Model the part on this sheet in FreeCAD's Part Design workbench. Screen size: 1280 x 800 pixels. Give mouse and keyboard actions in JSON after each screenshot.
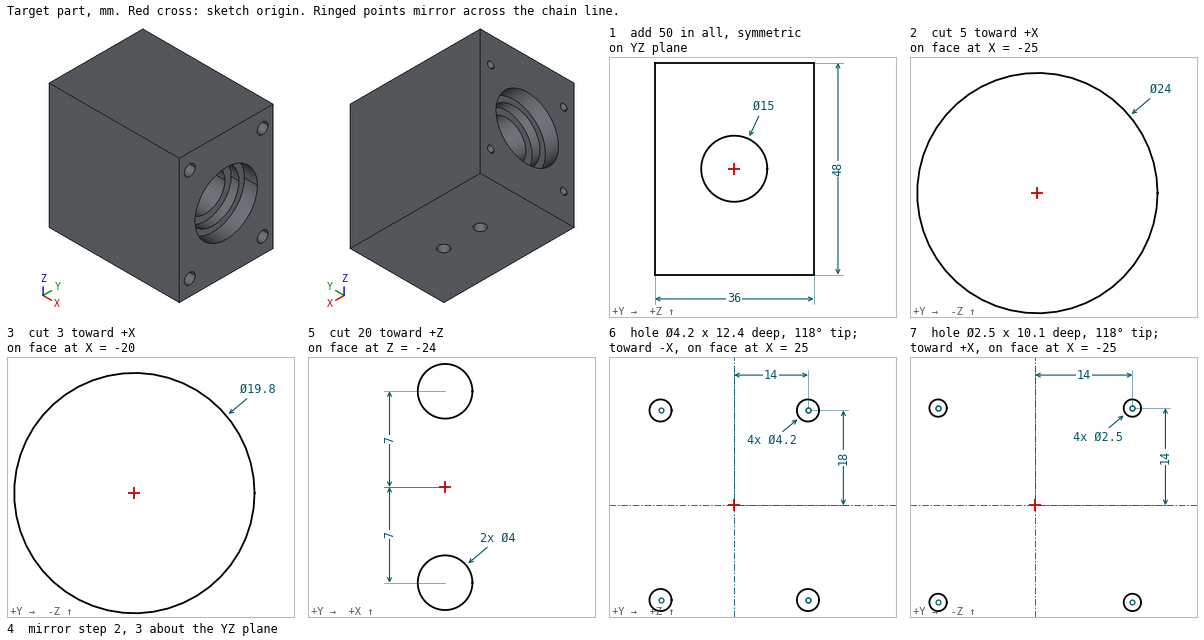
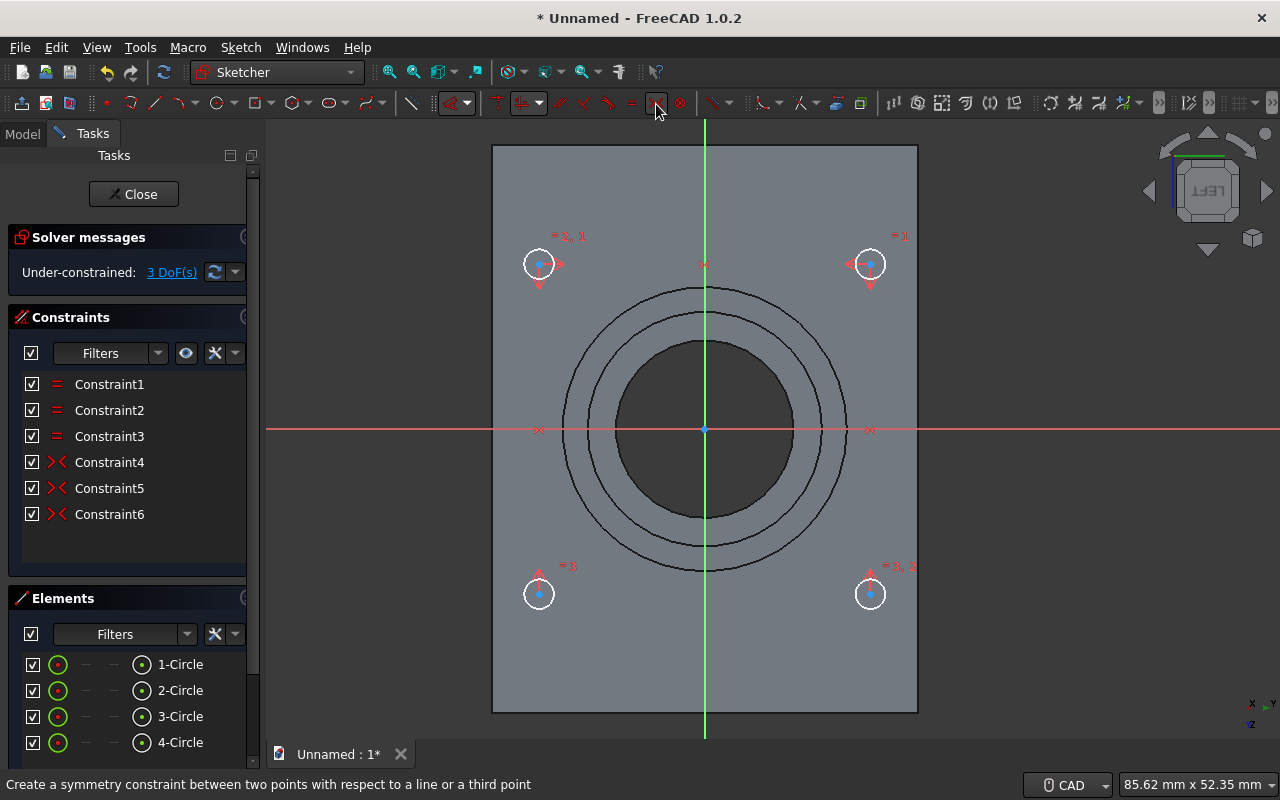
{"action": "scroll", "coordinate": [881, 254], "scroll_direction": "up", "scroll_amount": 2}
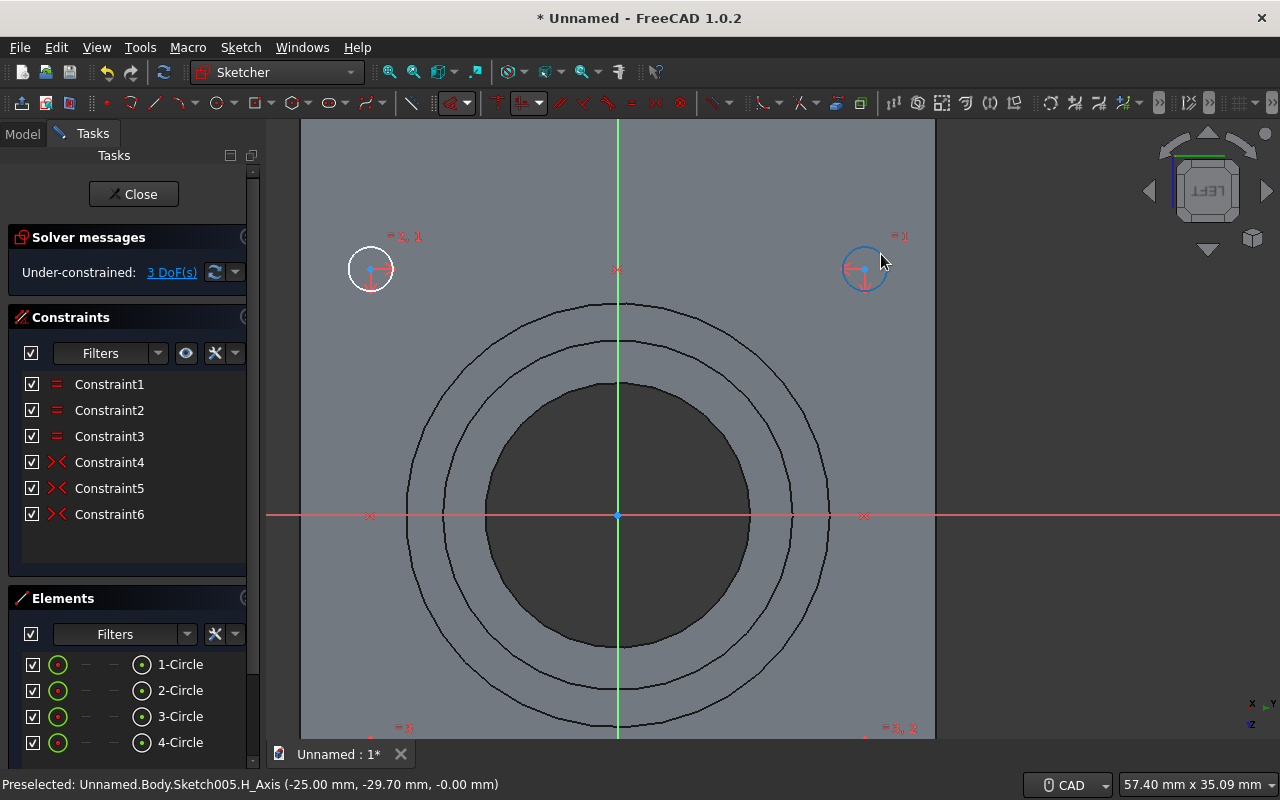
{"action": "left_click", "coordinate": [880, 254]}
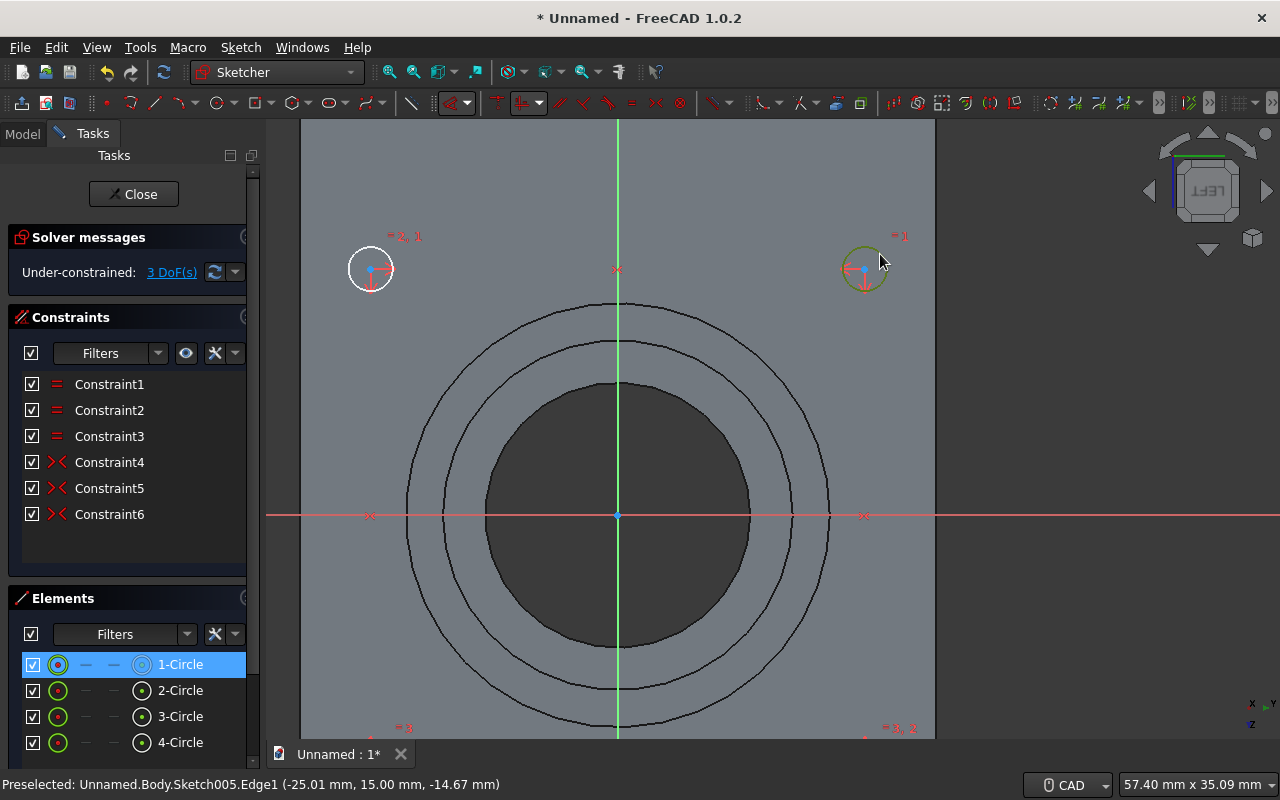
{"action": "key", "text": "k o"}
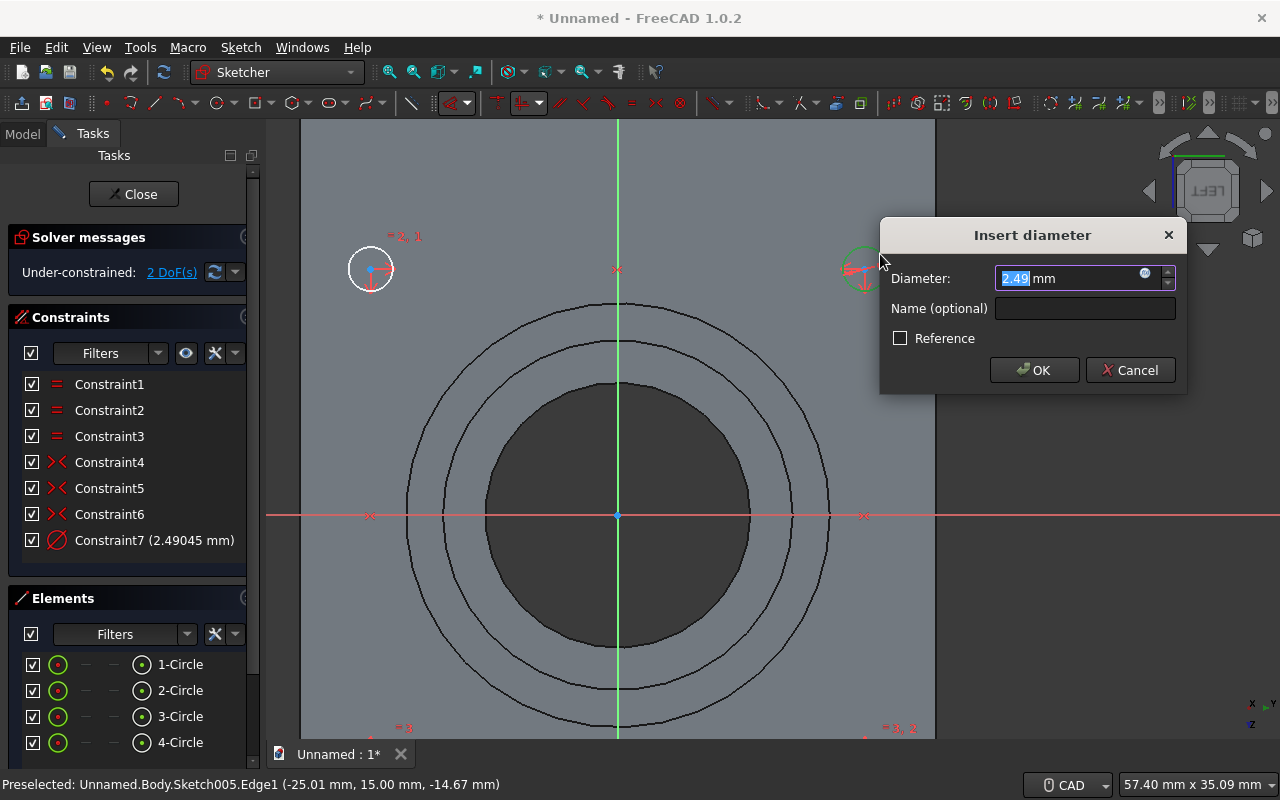
{"action": "type", "text": "2.5"}
{"action": "key", "text": "Return"}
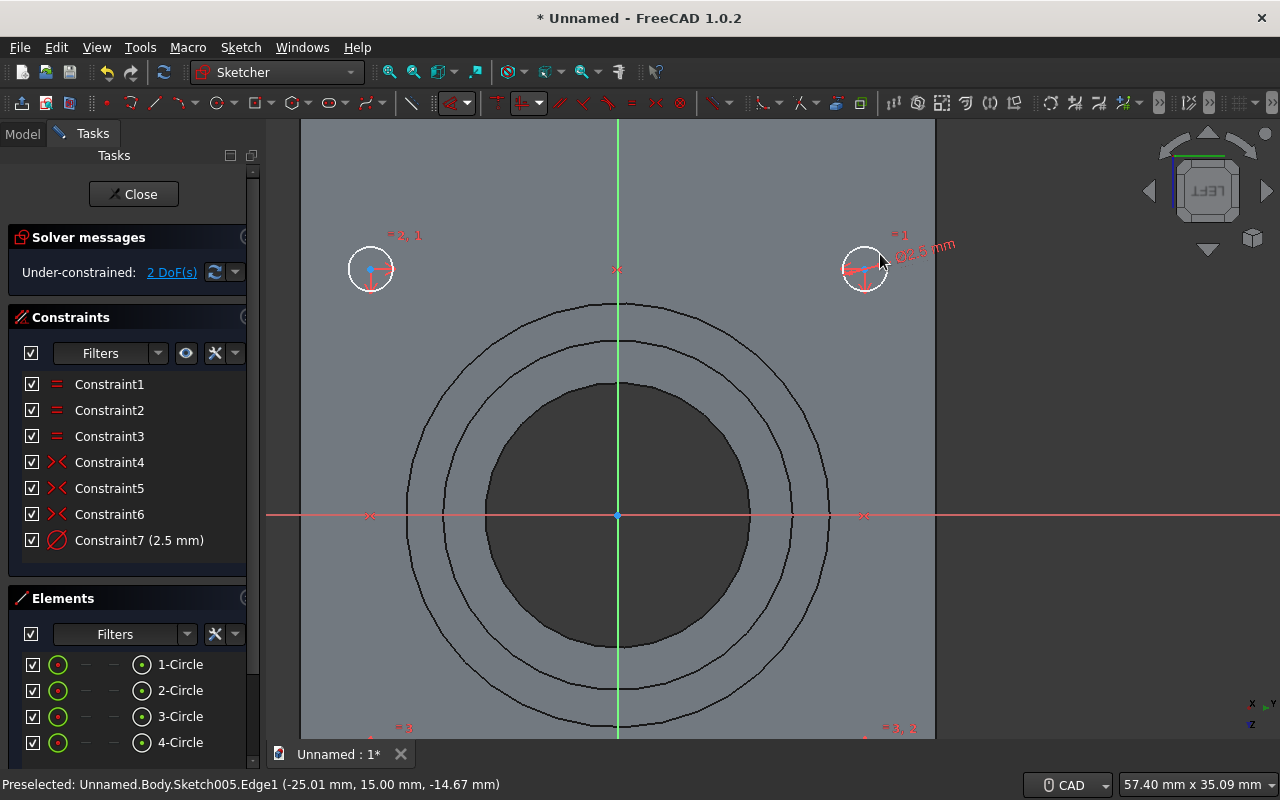
{"action": "left_click", "coordinate": [865, 269]}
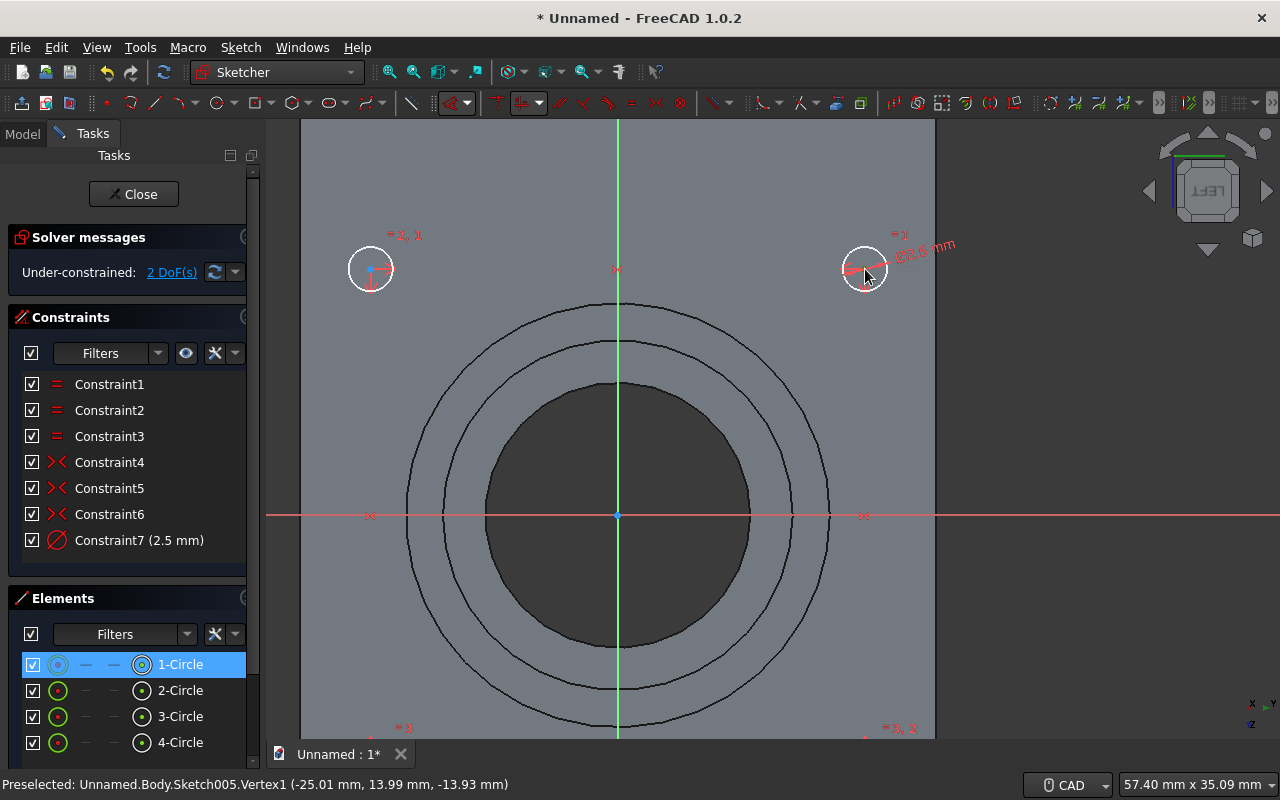
{"action": "left_click", "coordinate": [470, 104]}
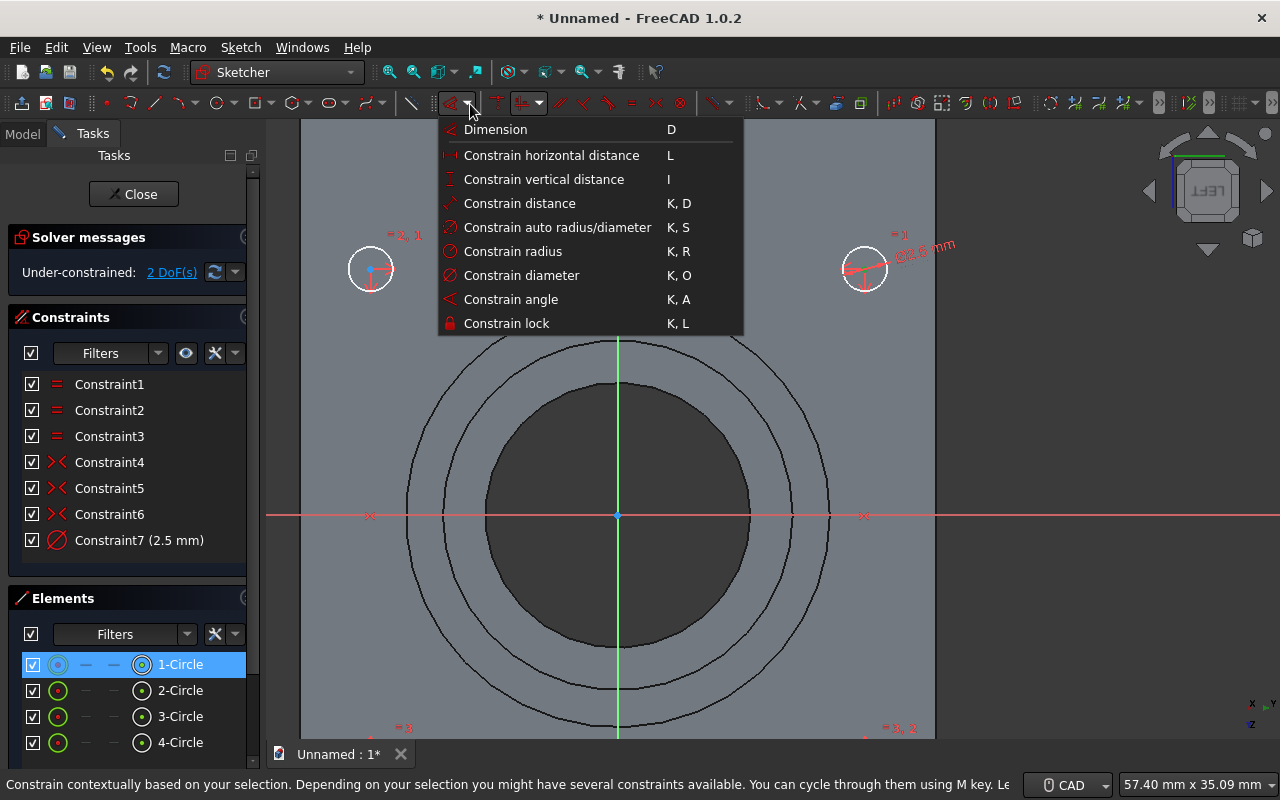
{"action": "left_click", "coordinate": [591, 155]}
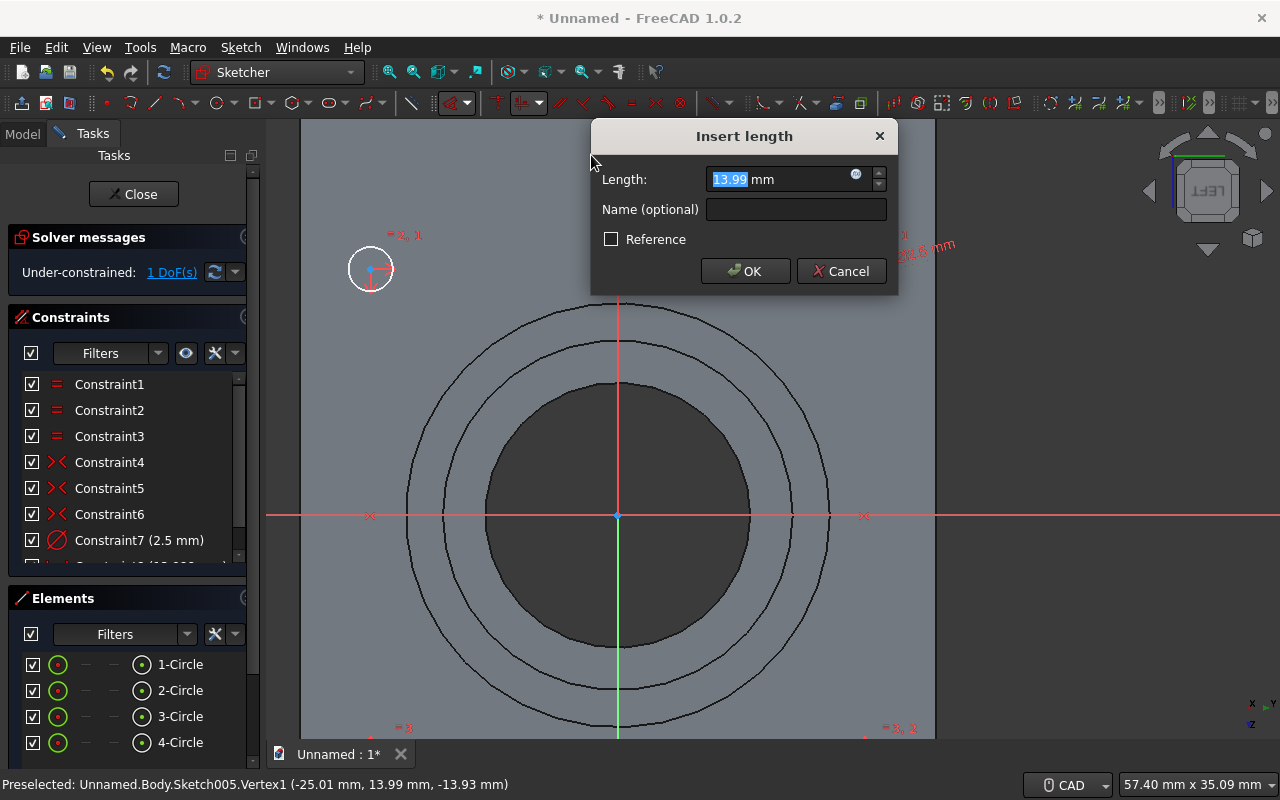
{"action": "type", "text": "14"}
{"action": "key", "text": "Return"}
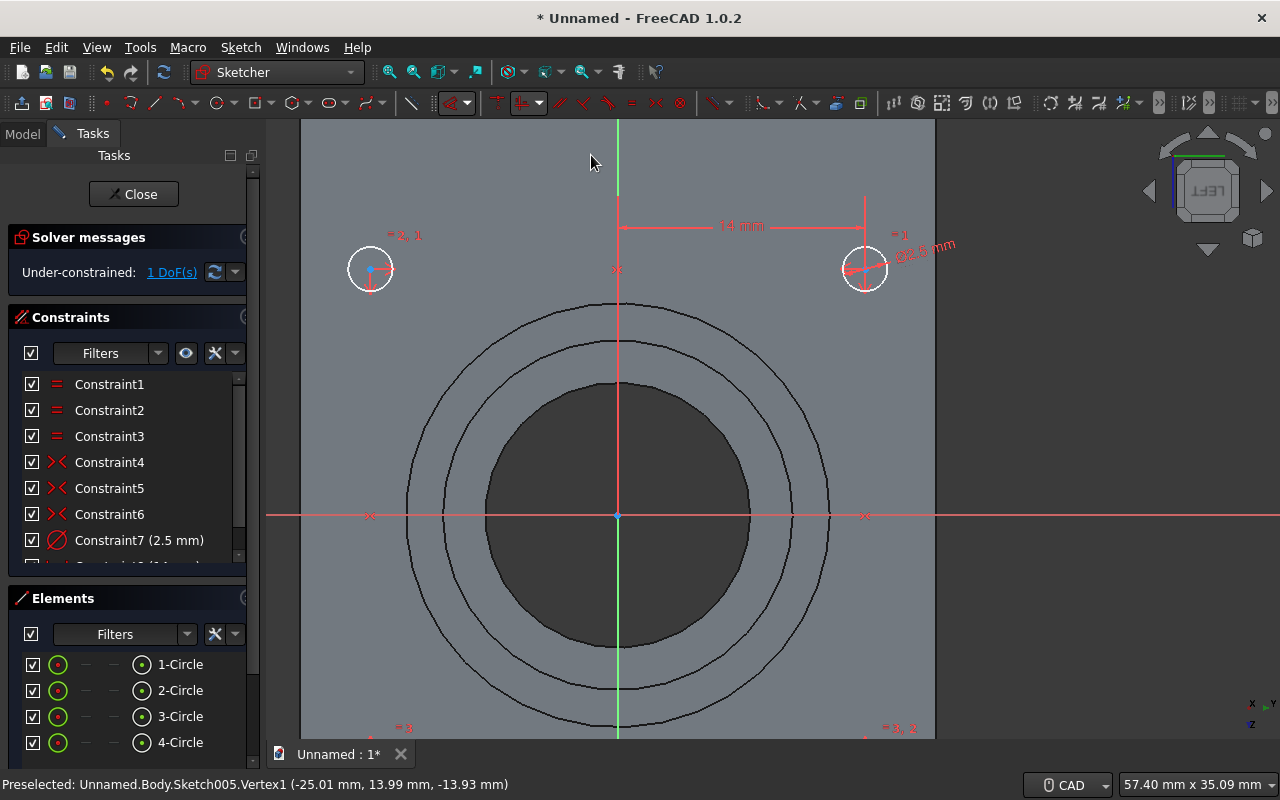
{"action": "left_click", "coordinate": [865, 269]}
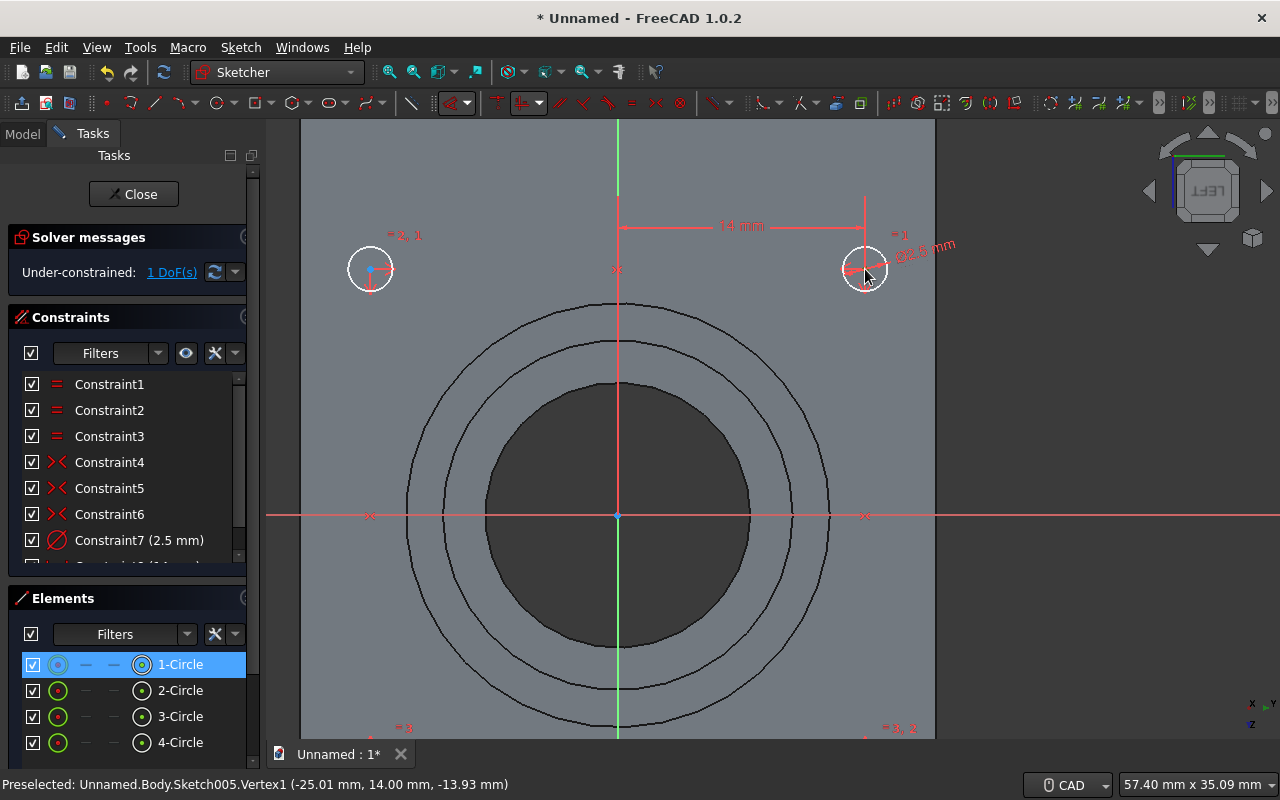
{"action": "left_click", "coordinate": [470, 104]}